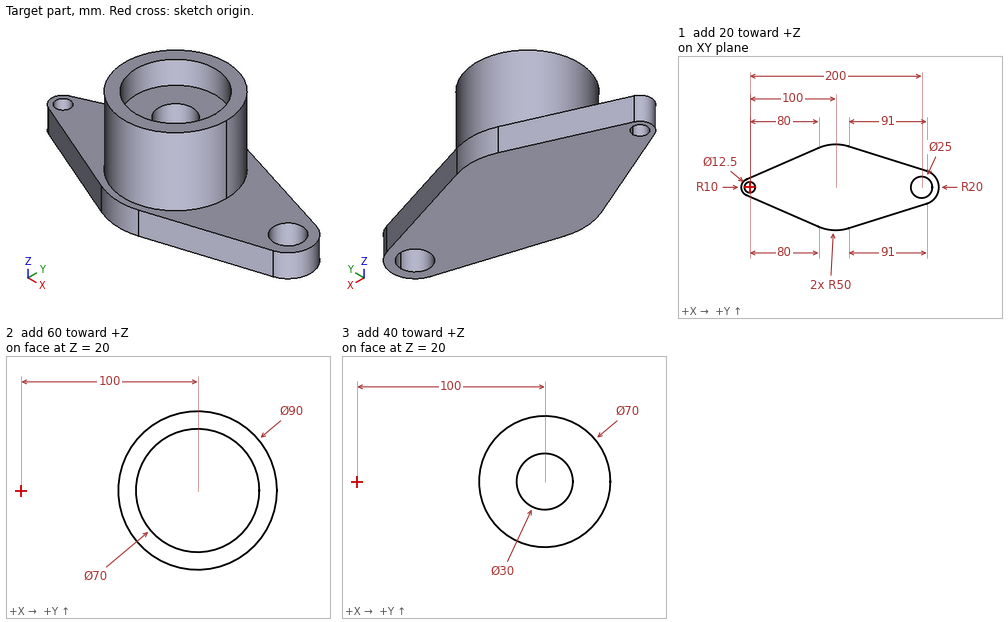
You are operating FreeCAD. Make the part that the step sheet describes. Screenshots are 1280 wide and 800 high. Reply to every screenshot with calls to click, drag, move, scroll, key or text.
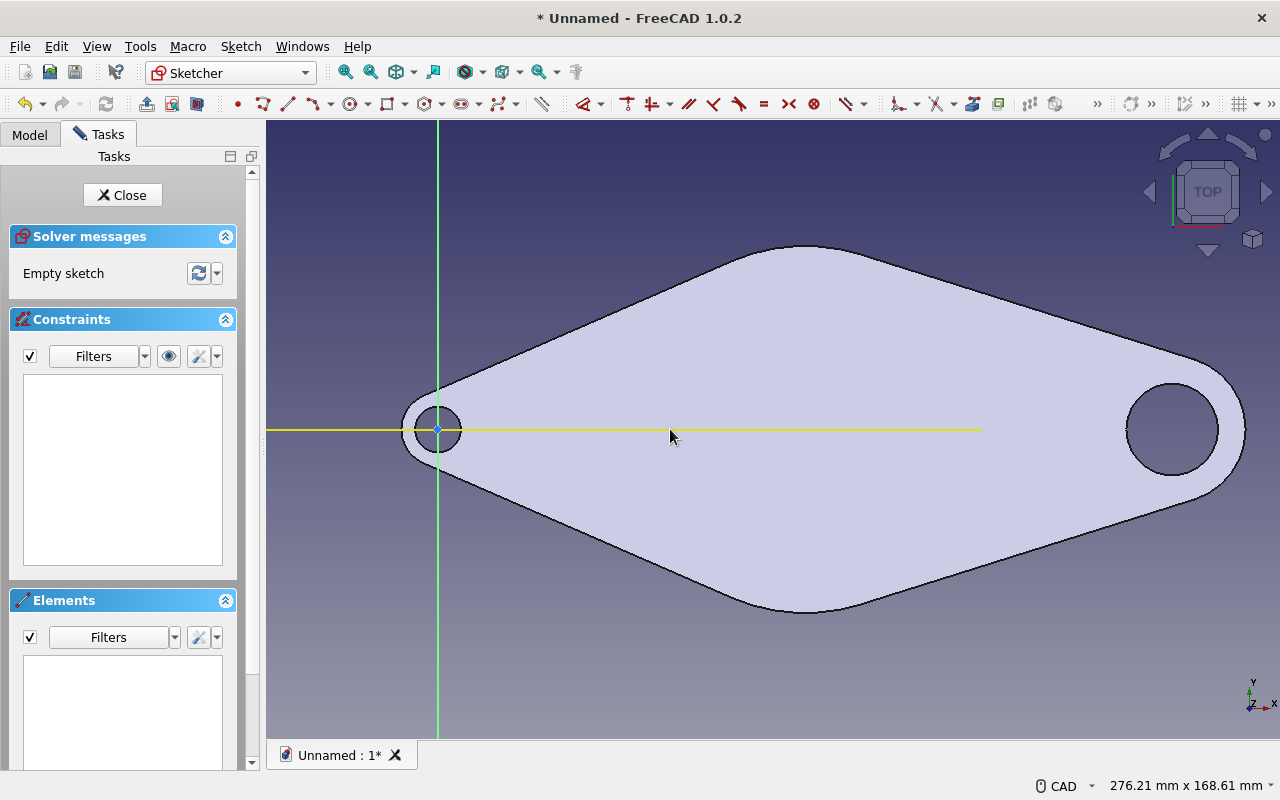
click(350, 104)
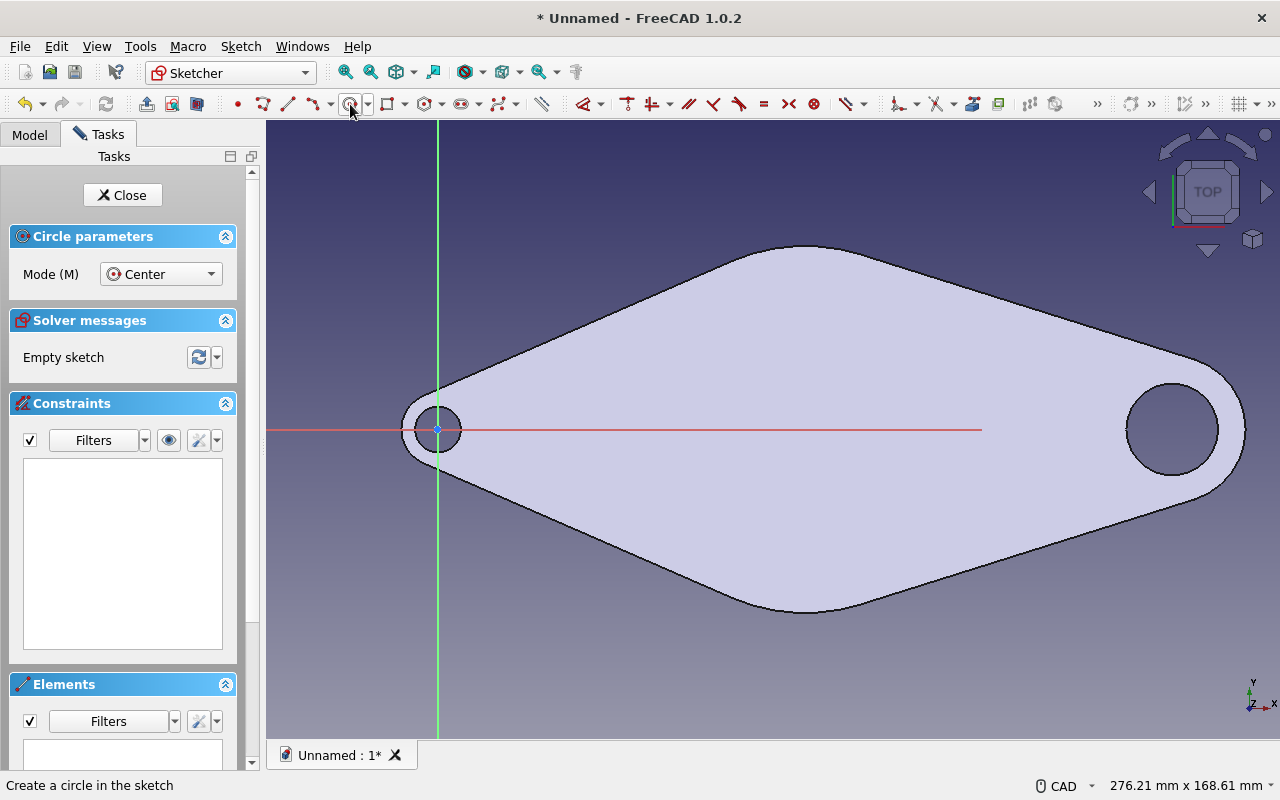
click(805, 430)
click(922, 313)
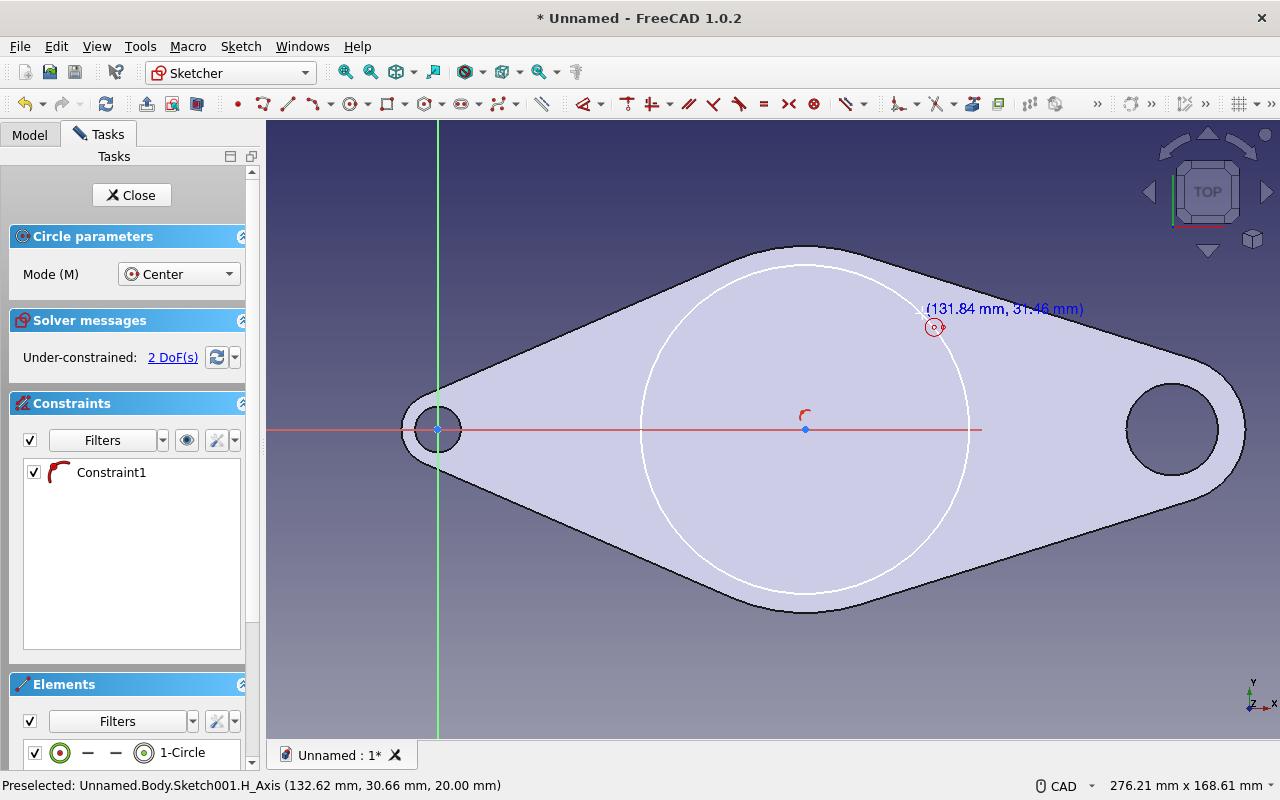
click(805, 430)
click(896, 339)
key(Escape)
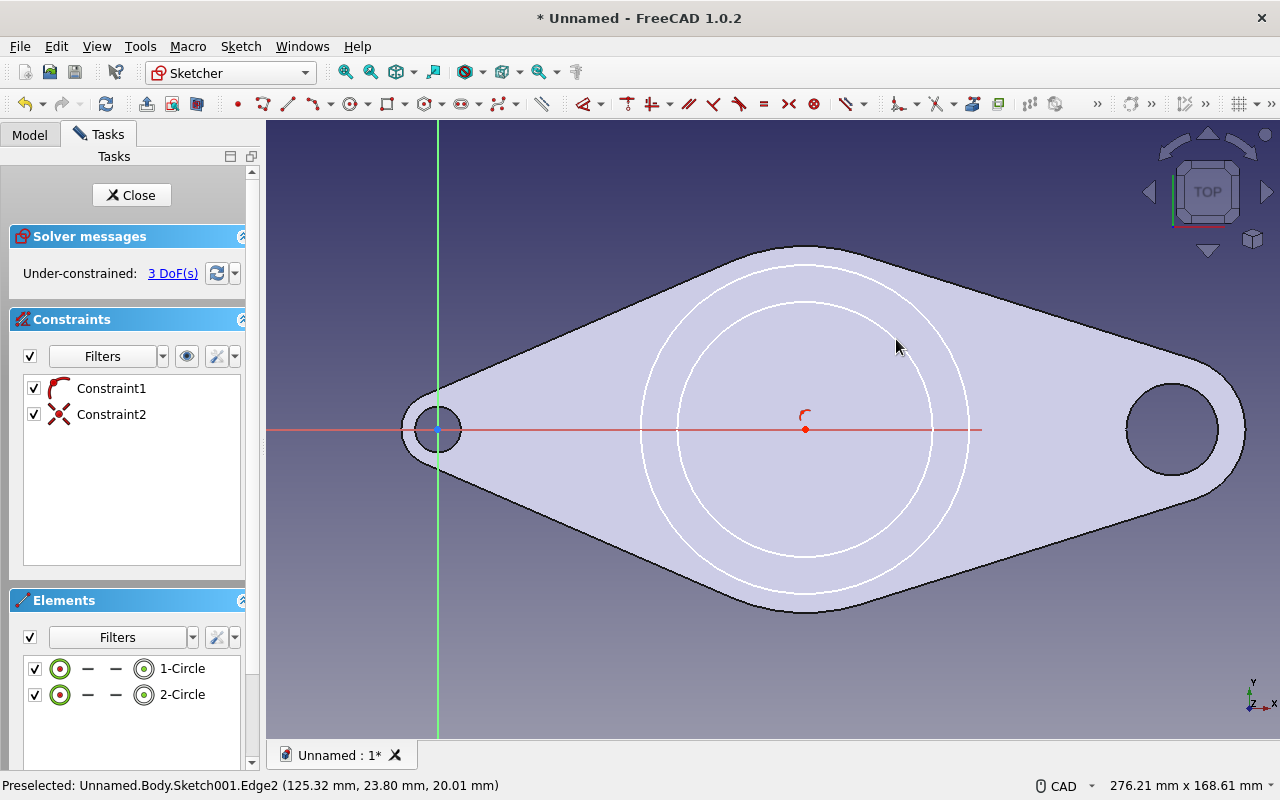
click(582, 104)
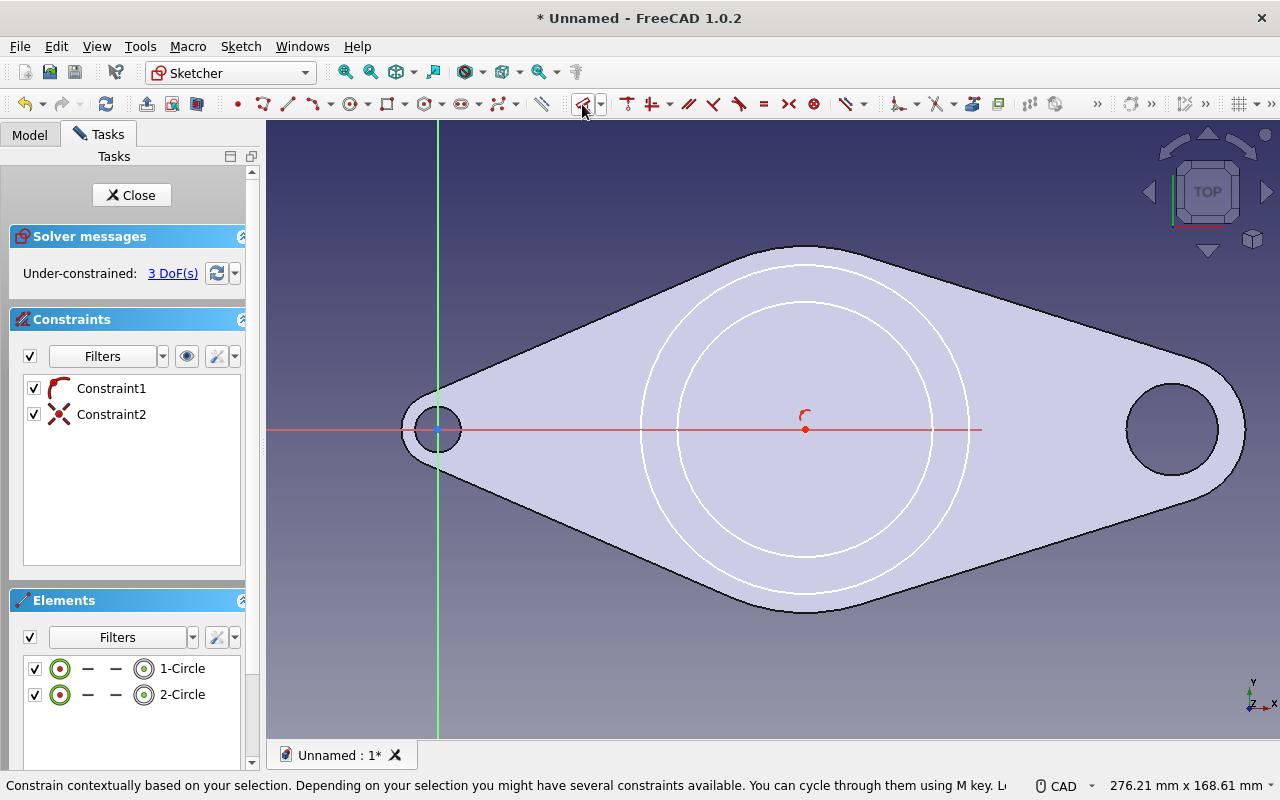
click(921, 313)
click(944, 290)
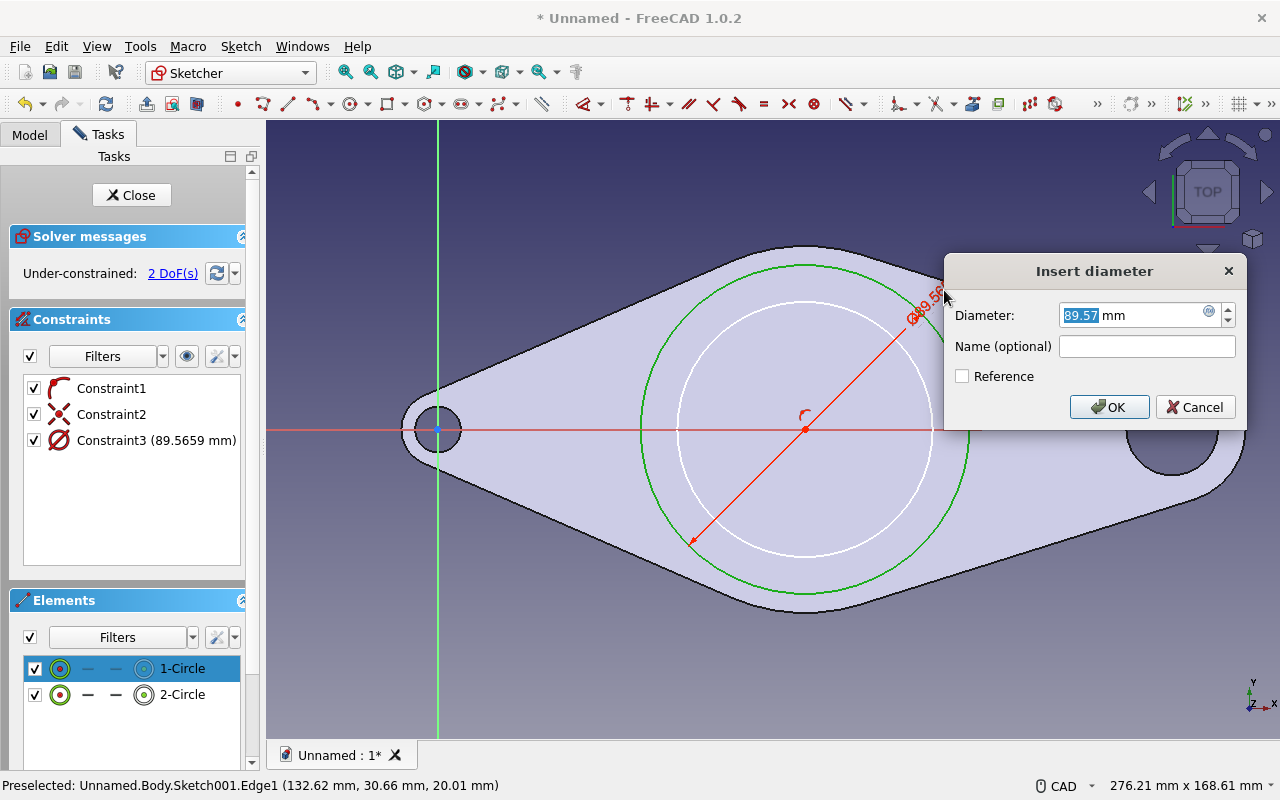
text(90)
key(Return)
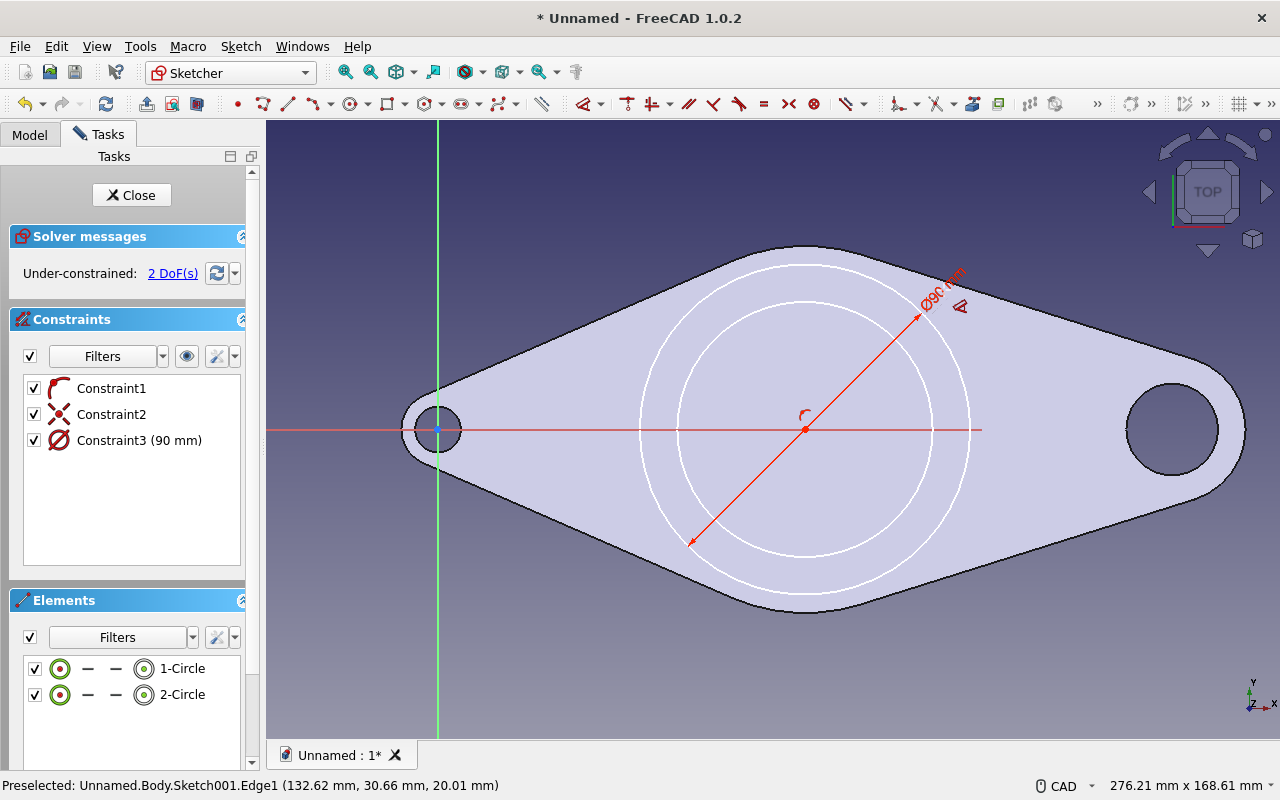
click(895, 339)
click(980, 378)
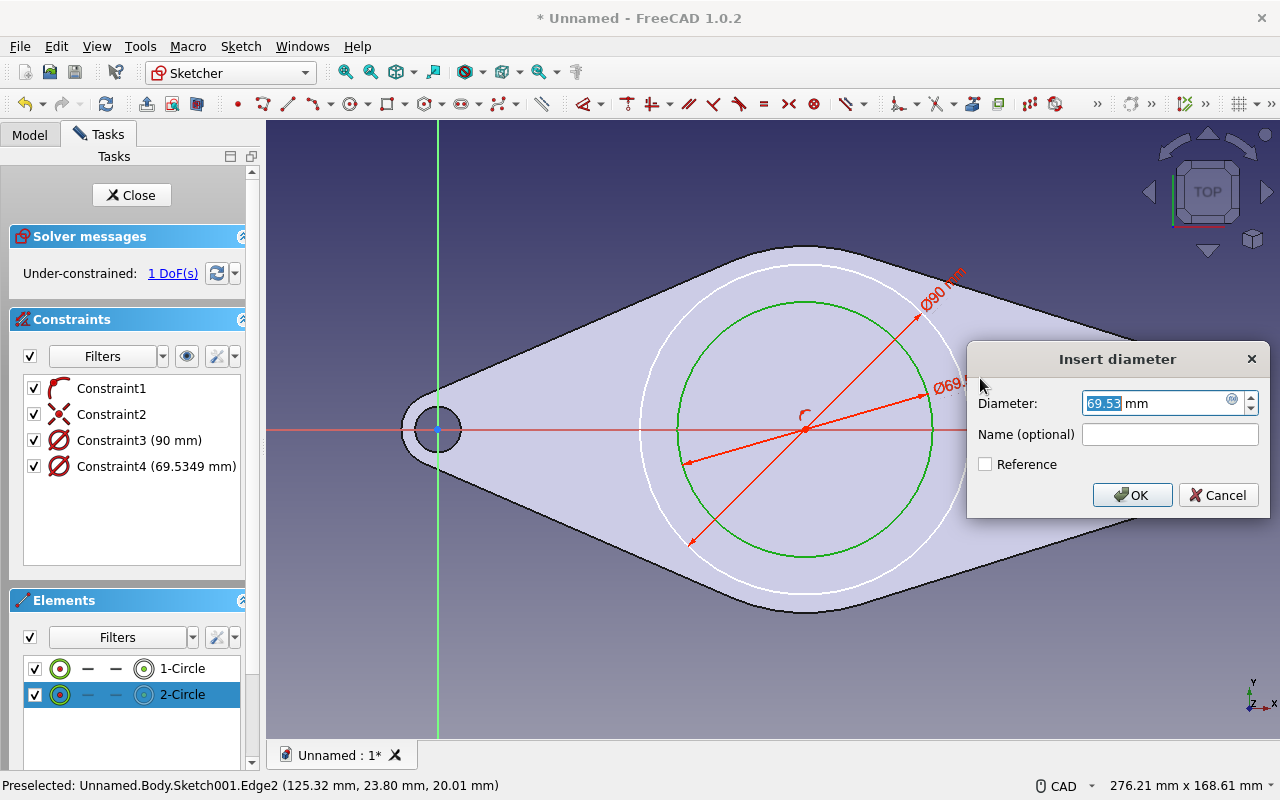
text(70)
key(Return)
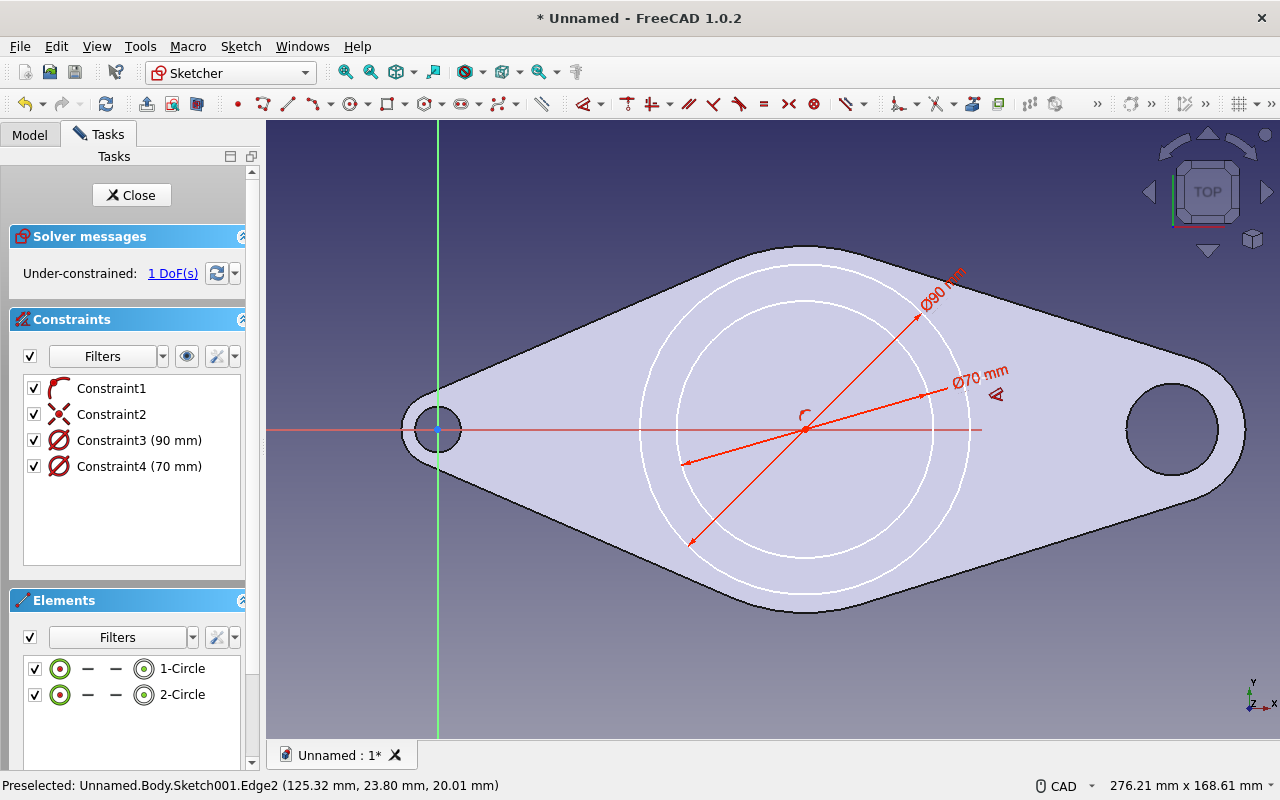
click(805, 430)
click(621, 464)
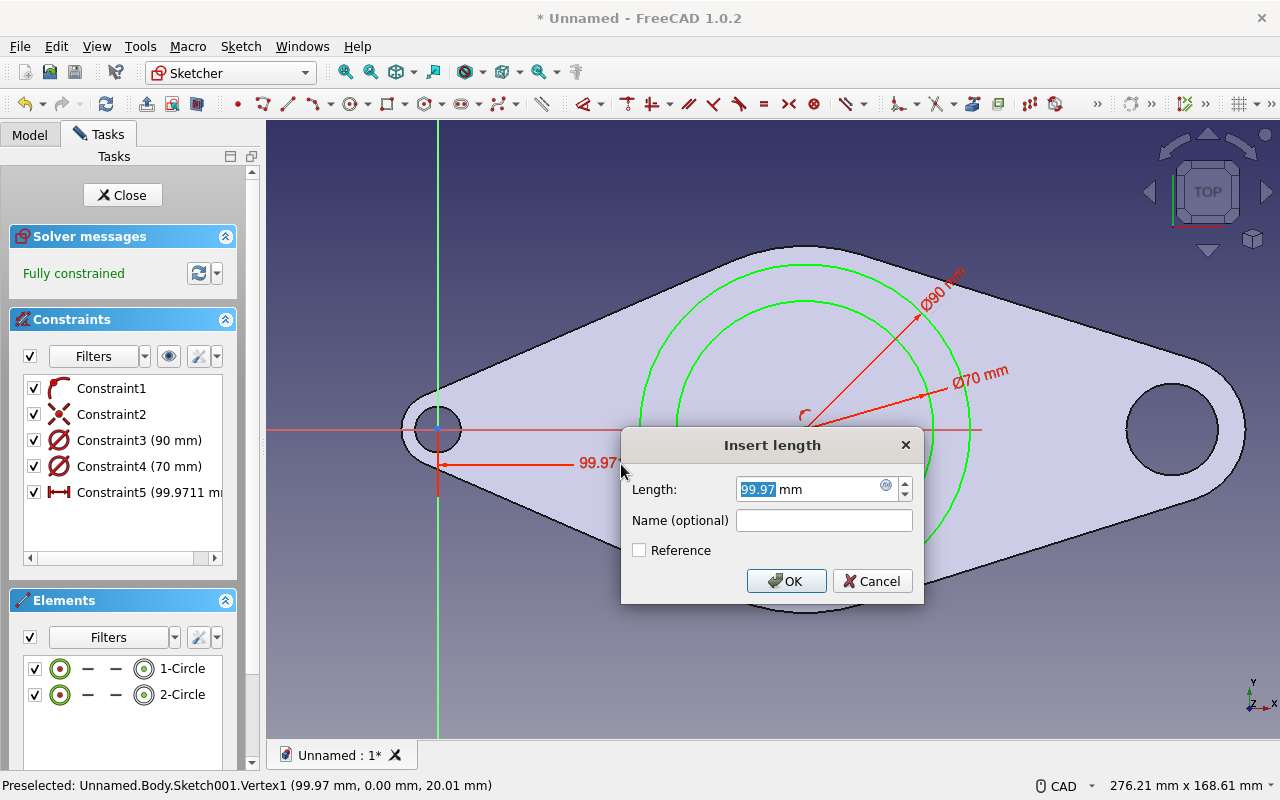
text(100)
key(Return)
key(Escape)